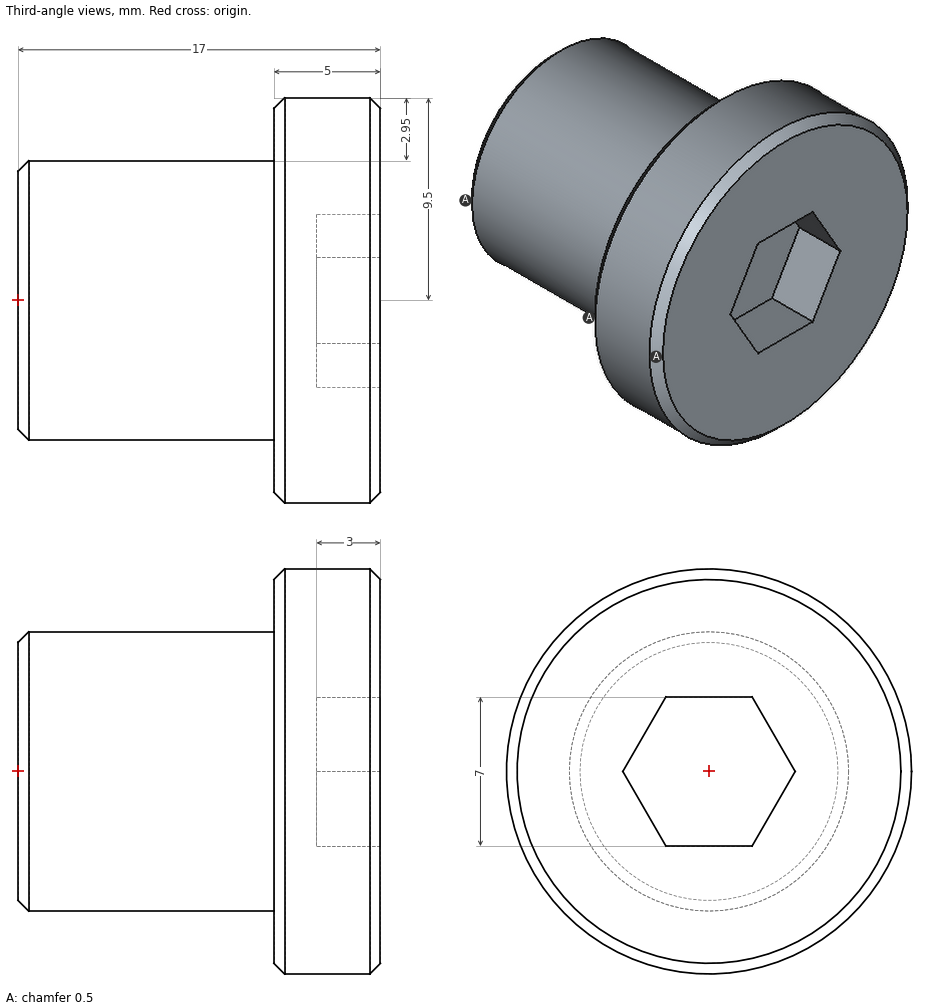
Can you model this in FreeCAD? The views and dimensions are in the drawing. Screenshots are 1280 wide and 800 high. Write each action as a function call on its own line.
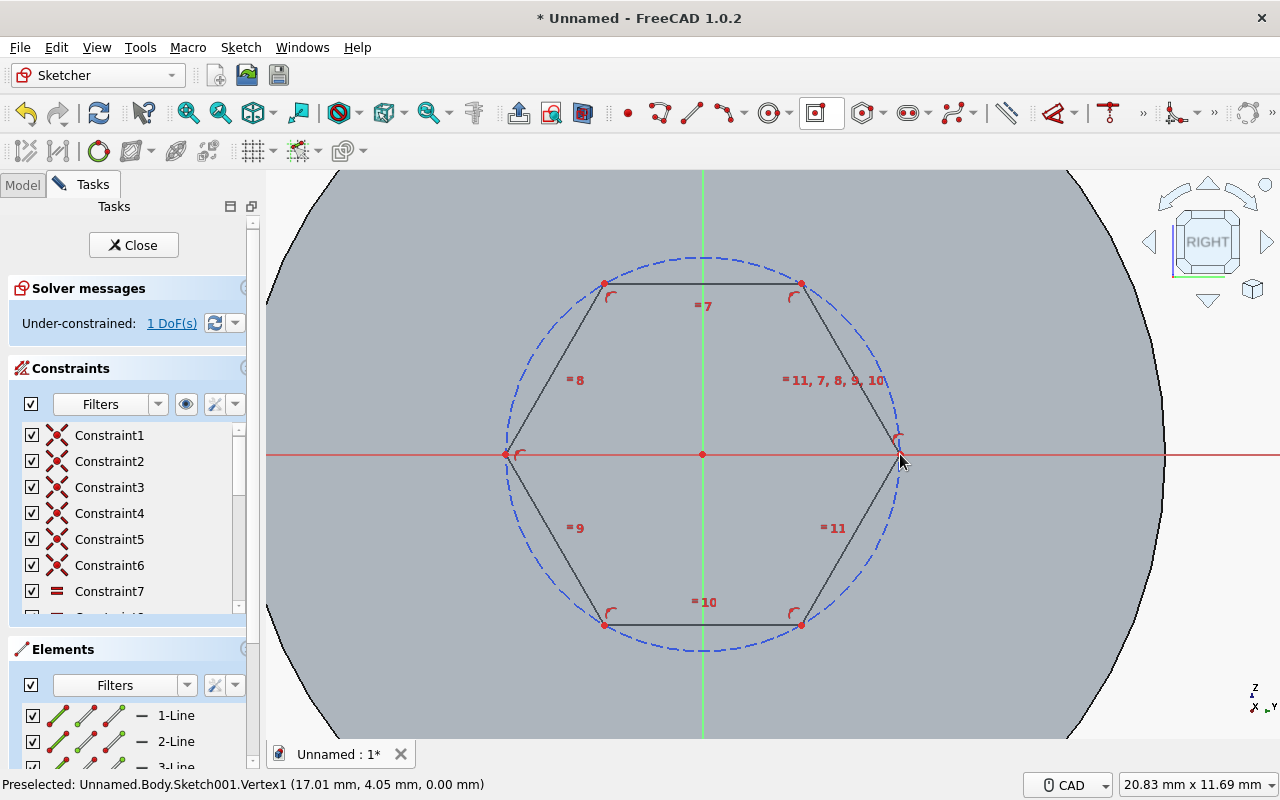
click(1054, 114)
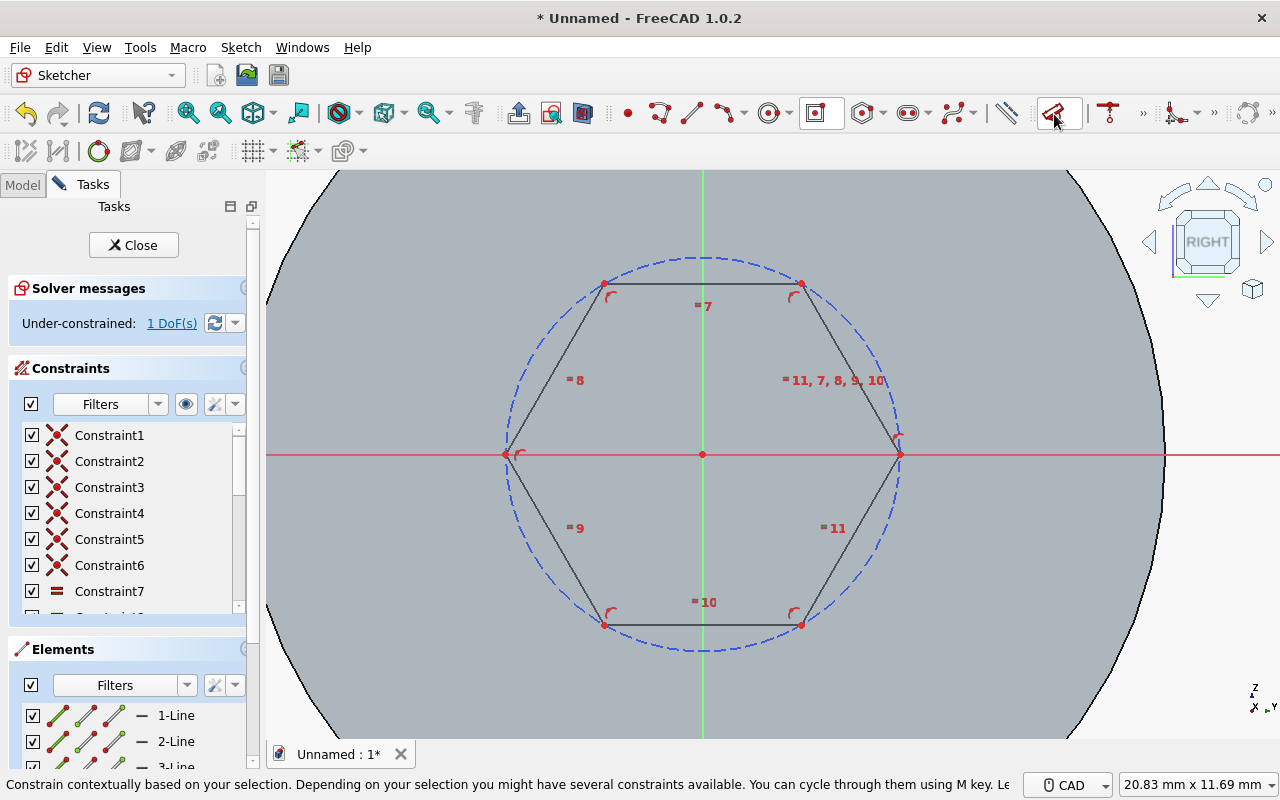
click(604, 625)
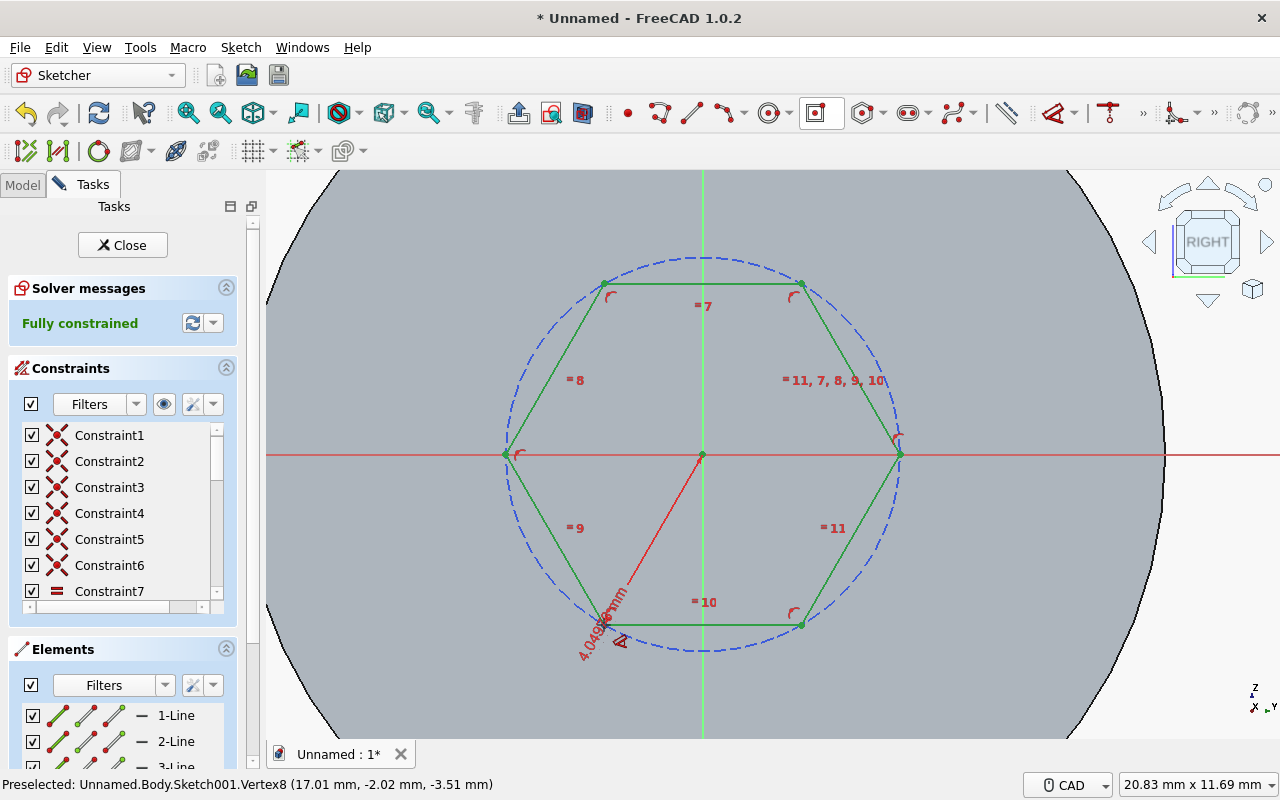
click(801, 284)
click(835, 376)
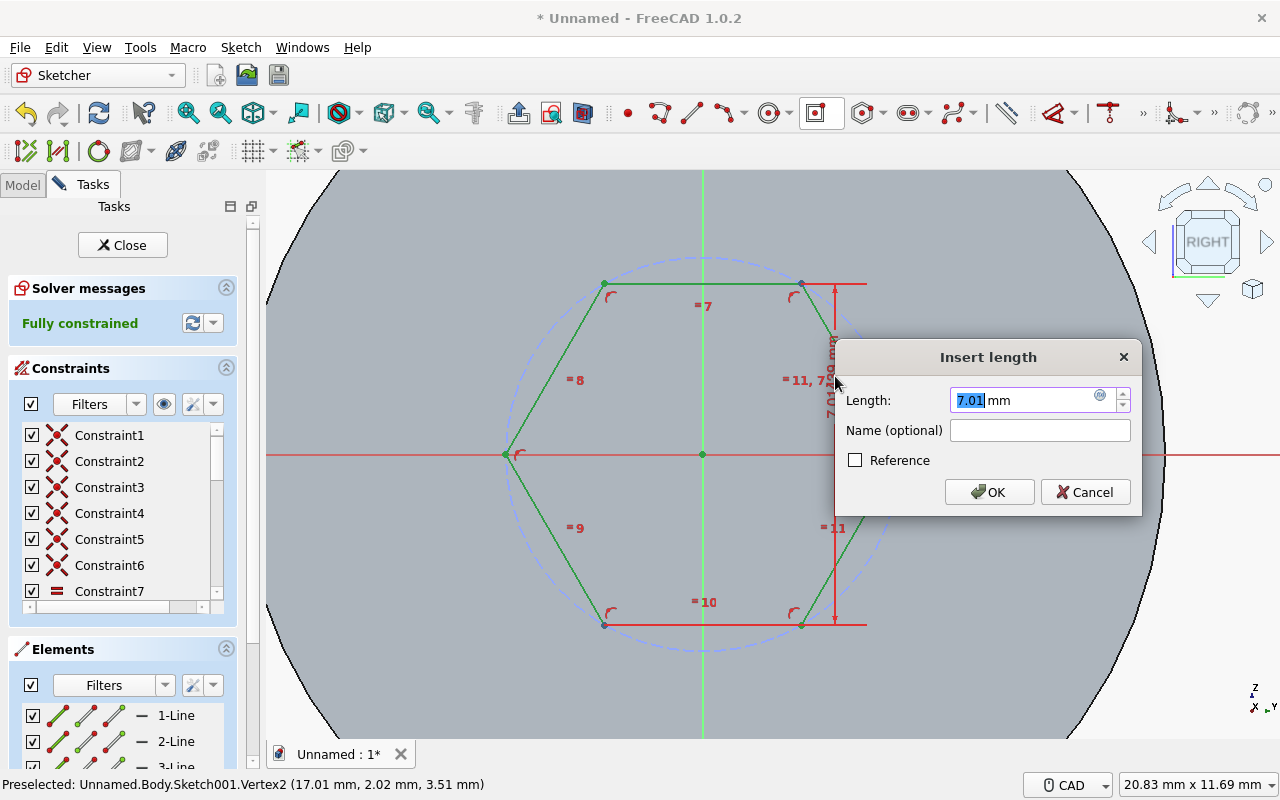
text(7)
key(Return)
key(Escape)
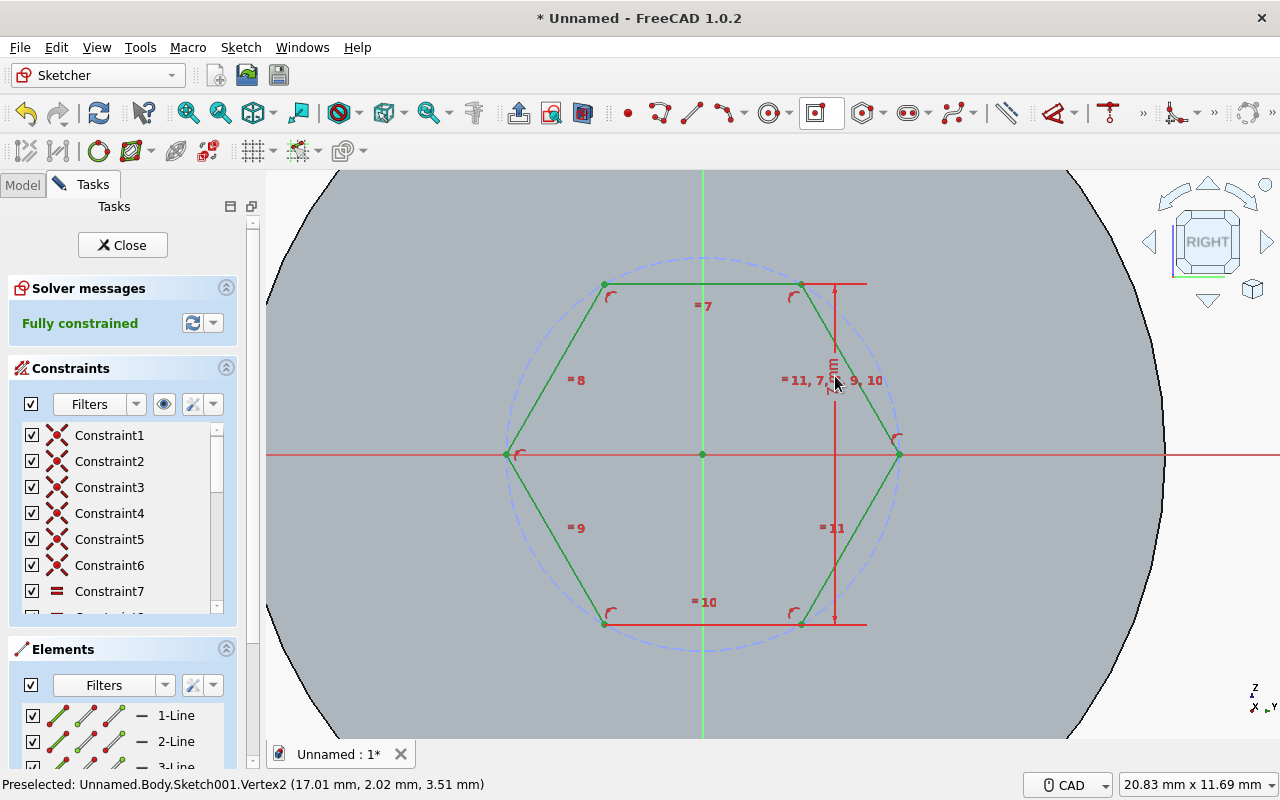
click(123, 245)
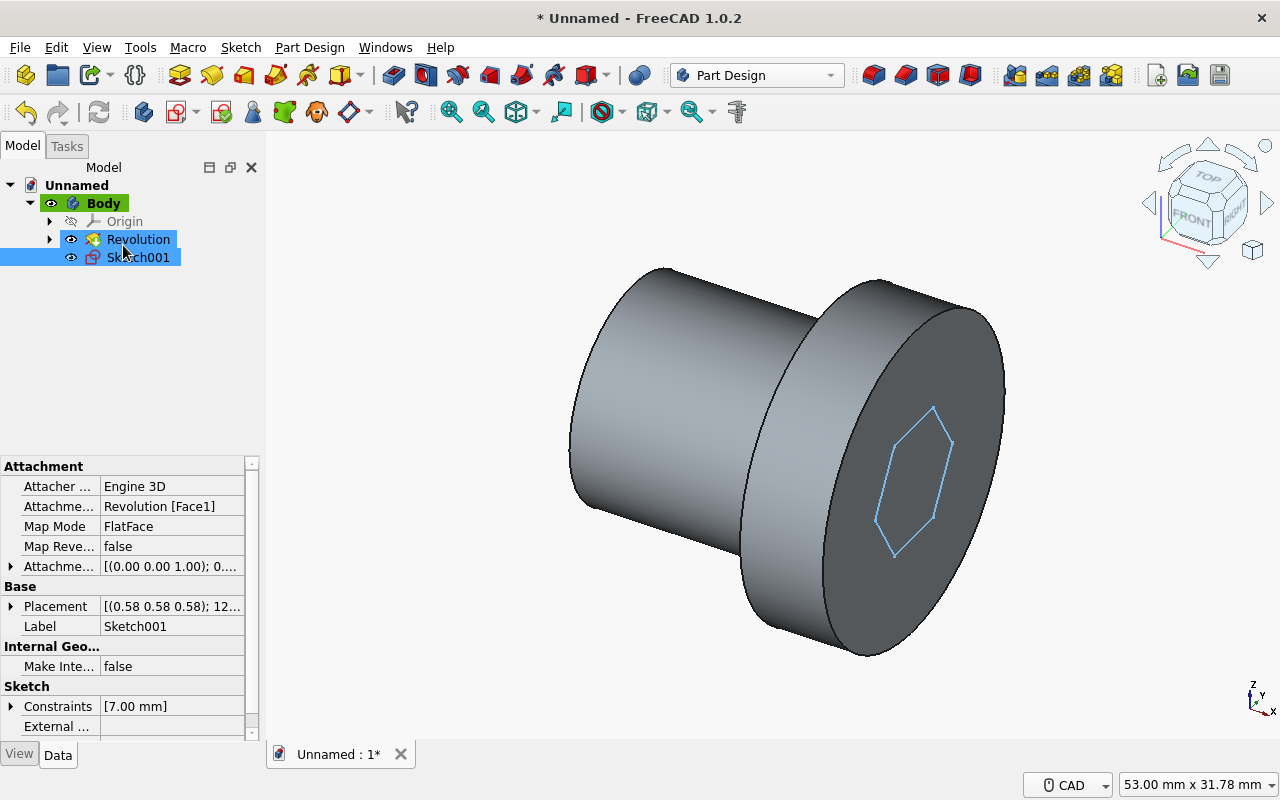
click(394, 76)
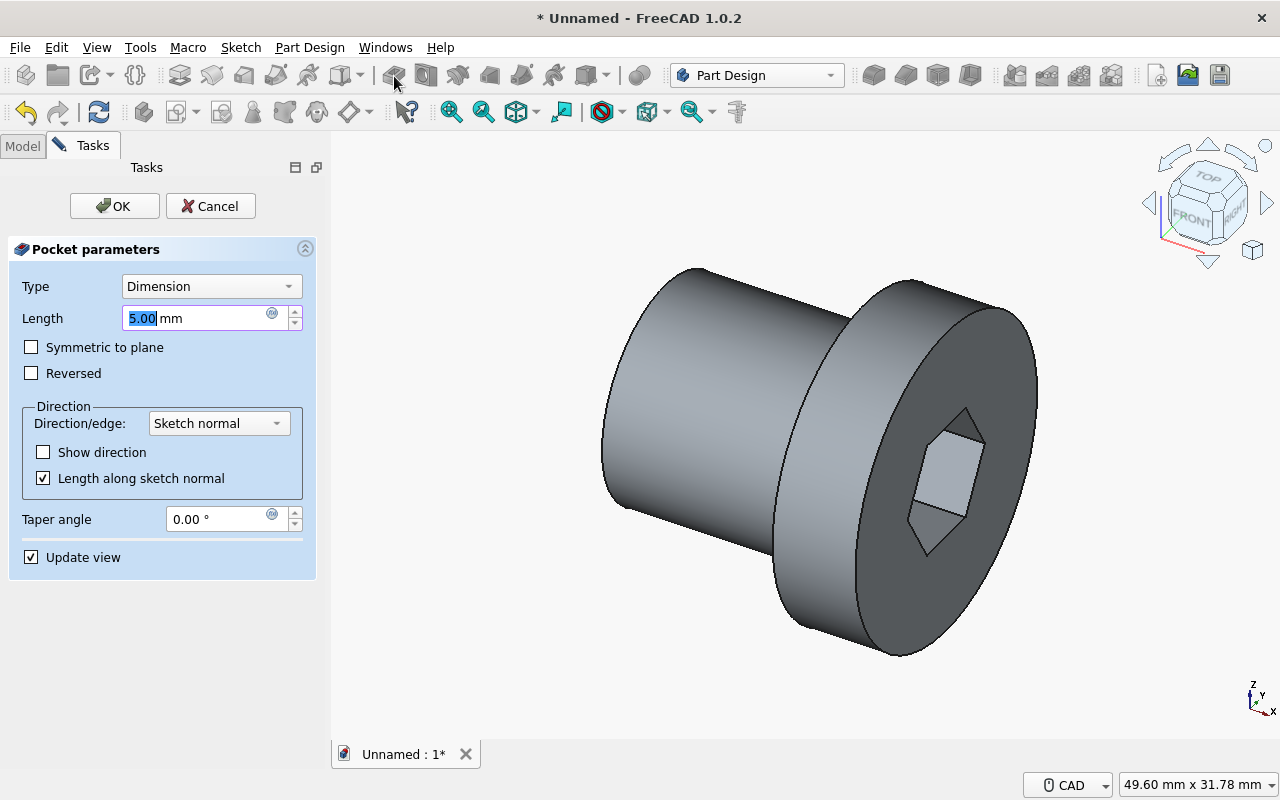
text(3)
key(Tab)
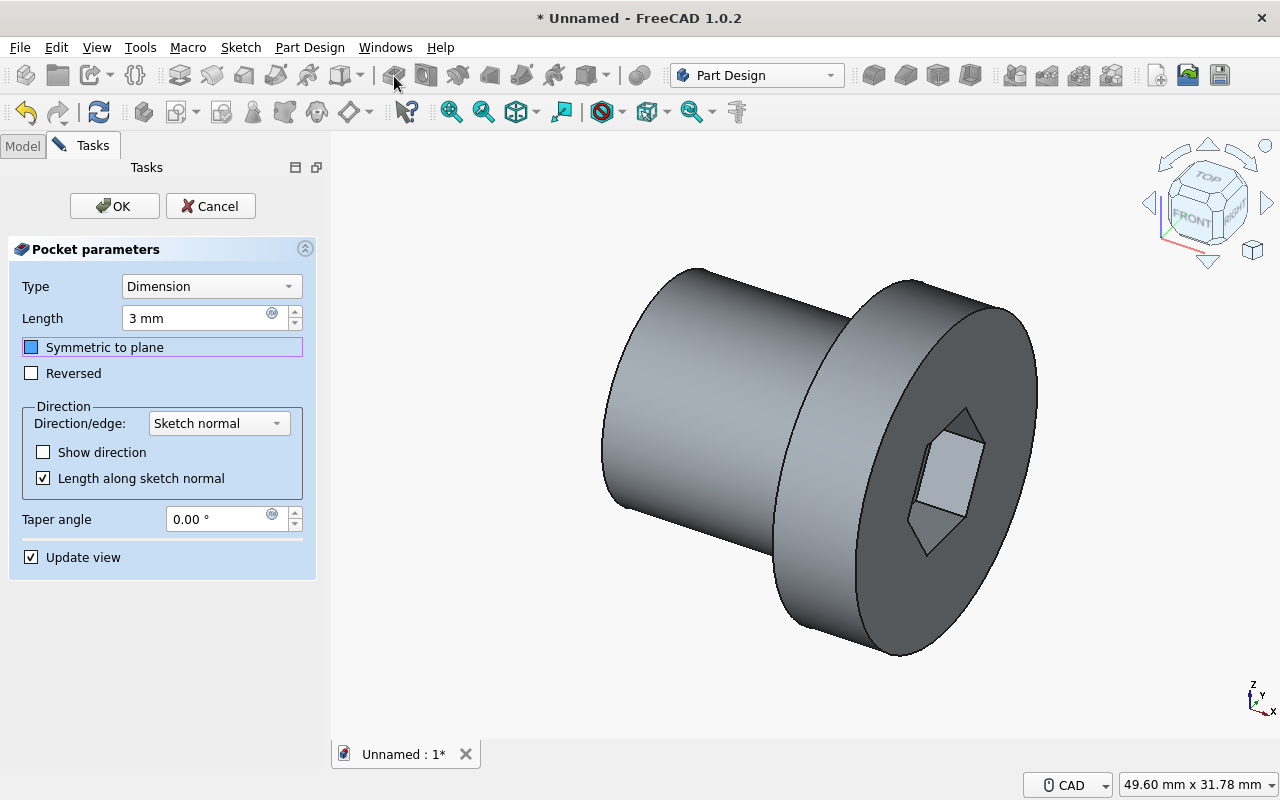
click(115, 206)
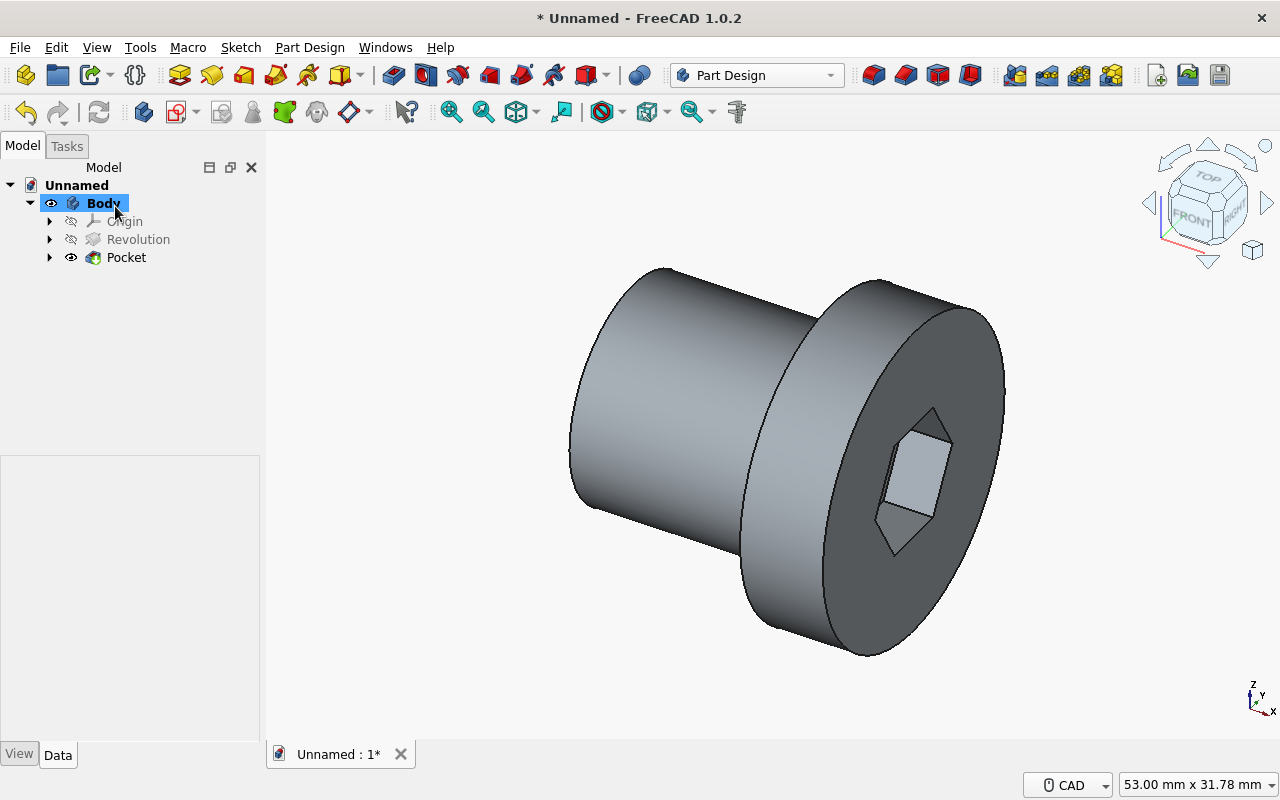
click(823, 571)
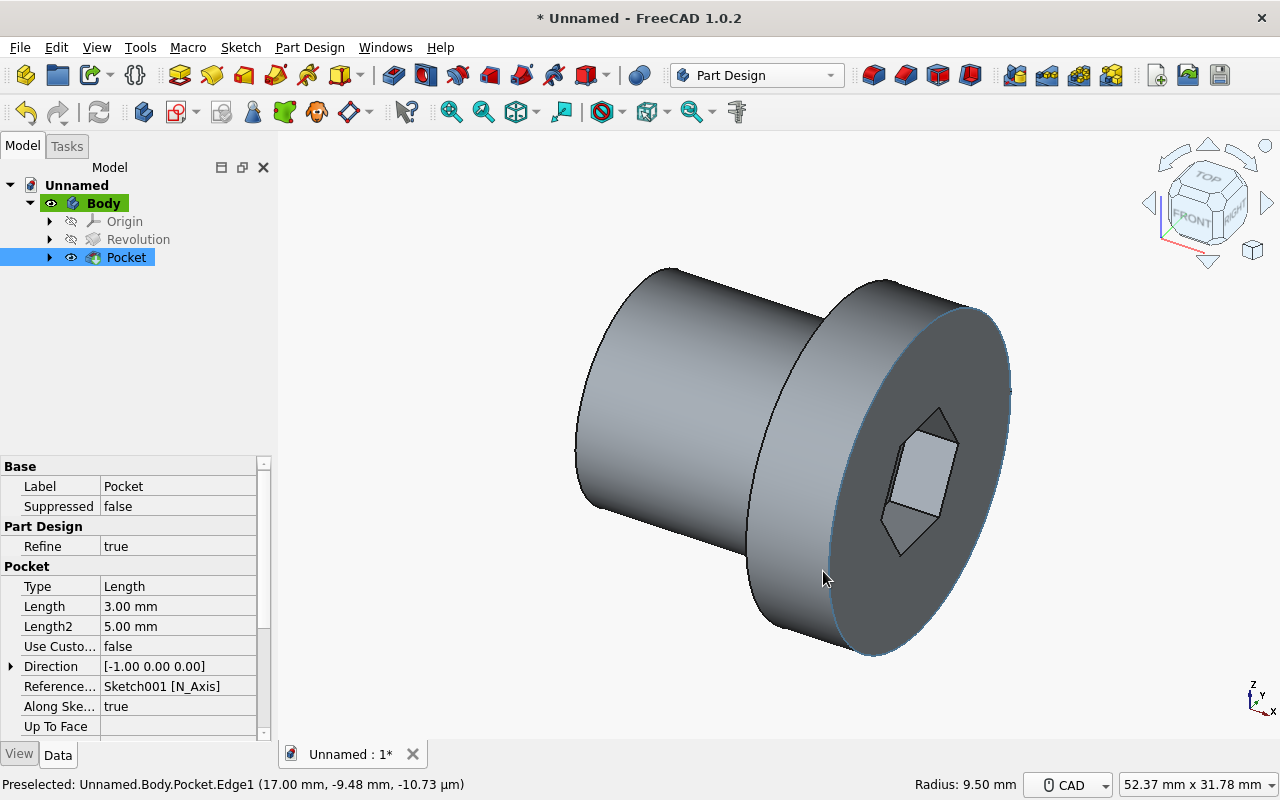
key(0)